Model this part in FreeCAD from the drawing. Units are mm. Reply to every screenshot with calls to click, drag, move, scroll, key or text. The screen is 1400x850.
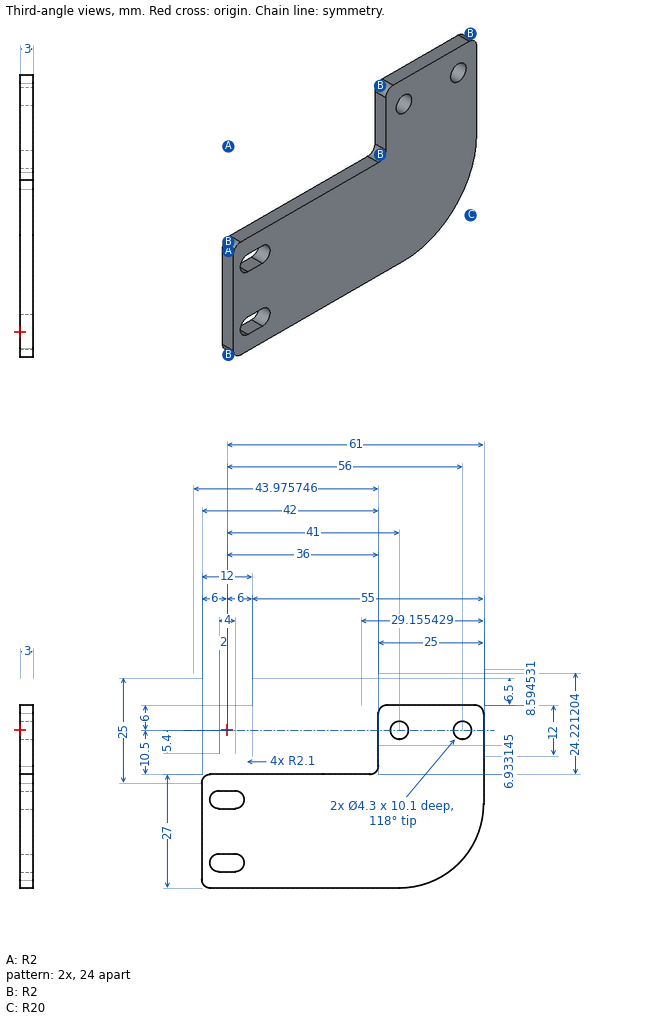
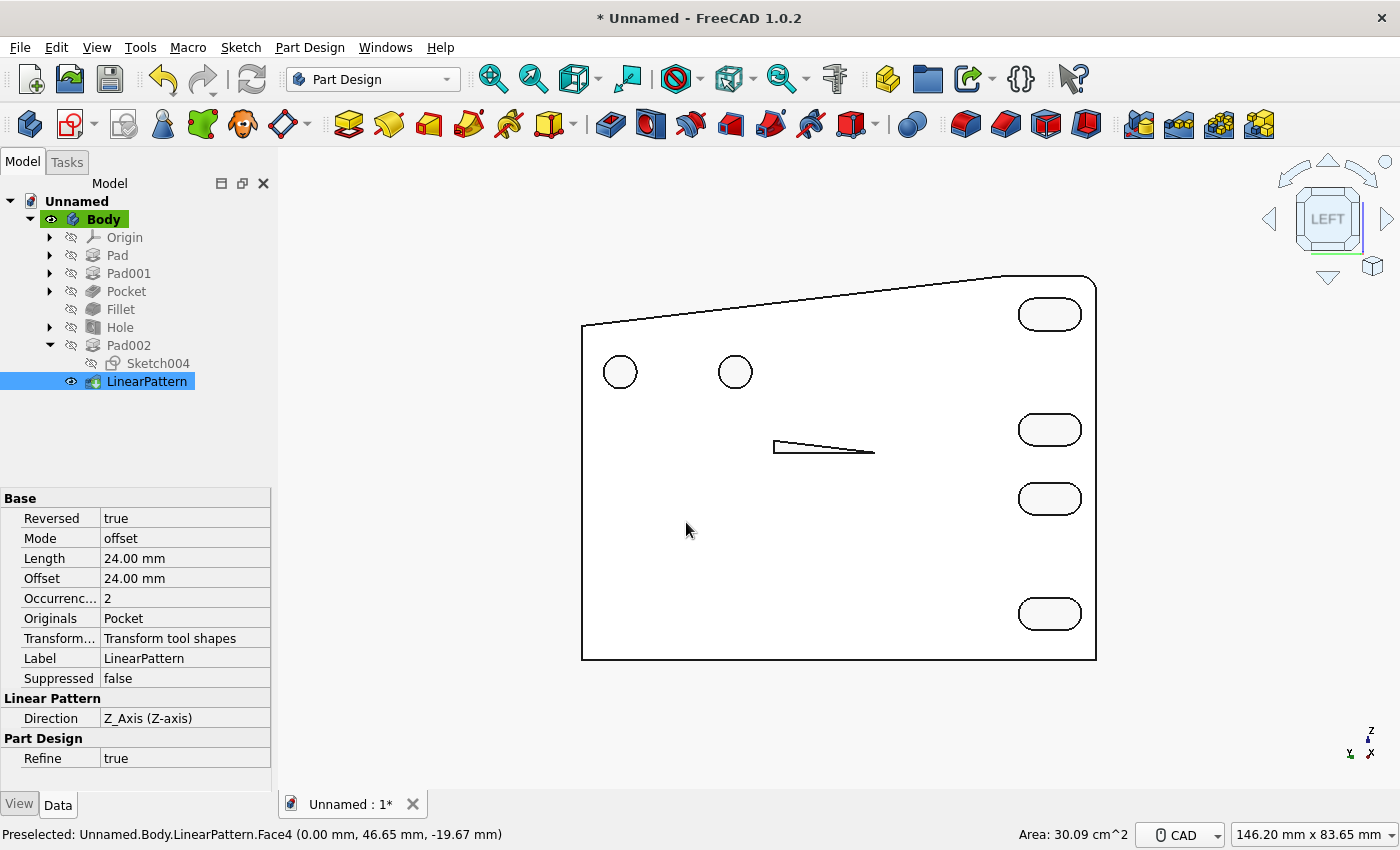
click(70, 124)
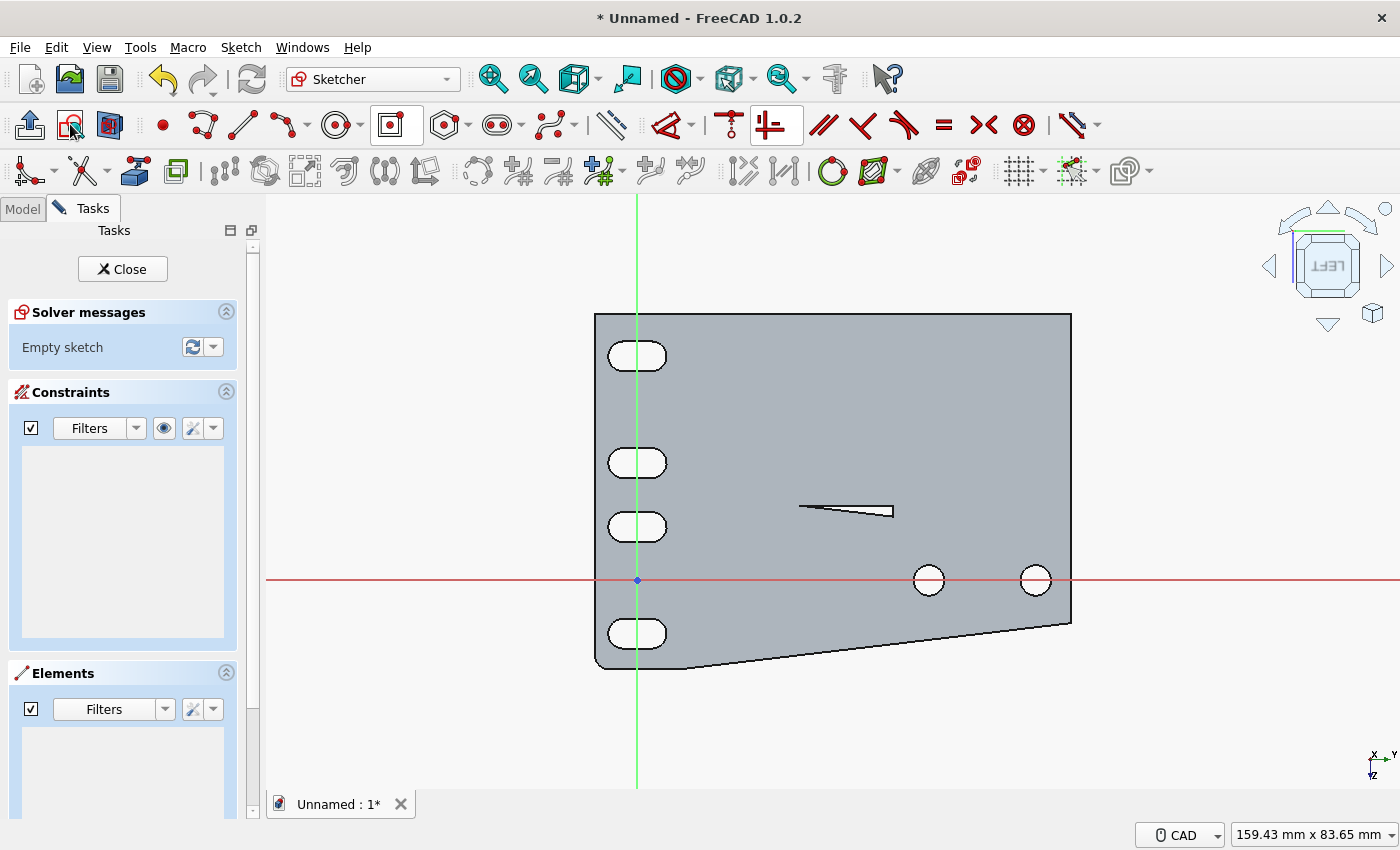
scroll(715, 674, up, 4)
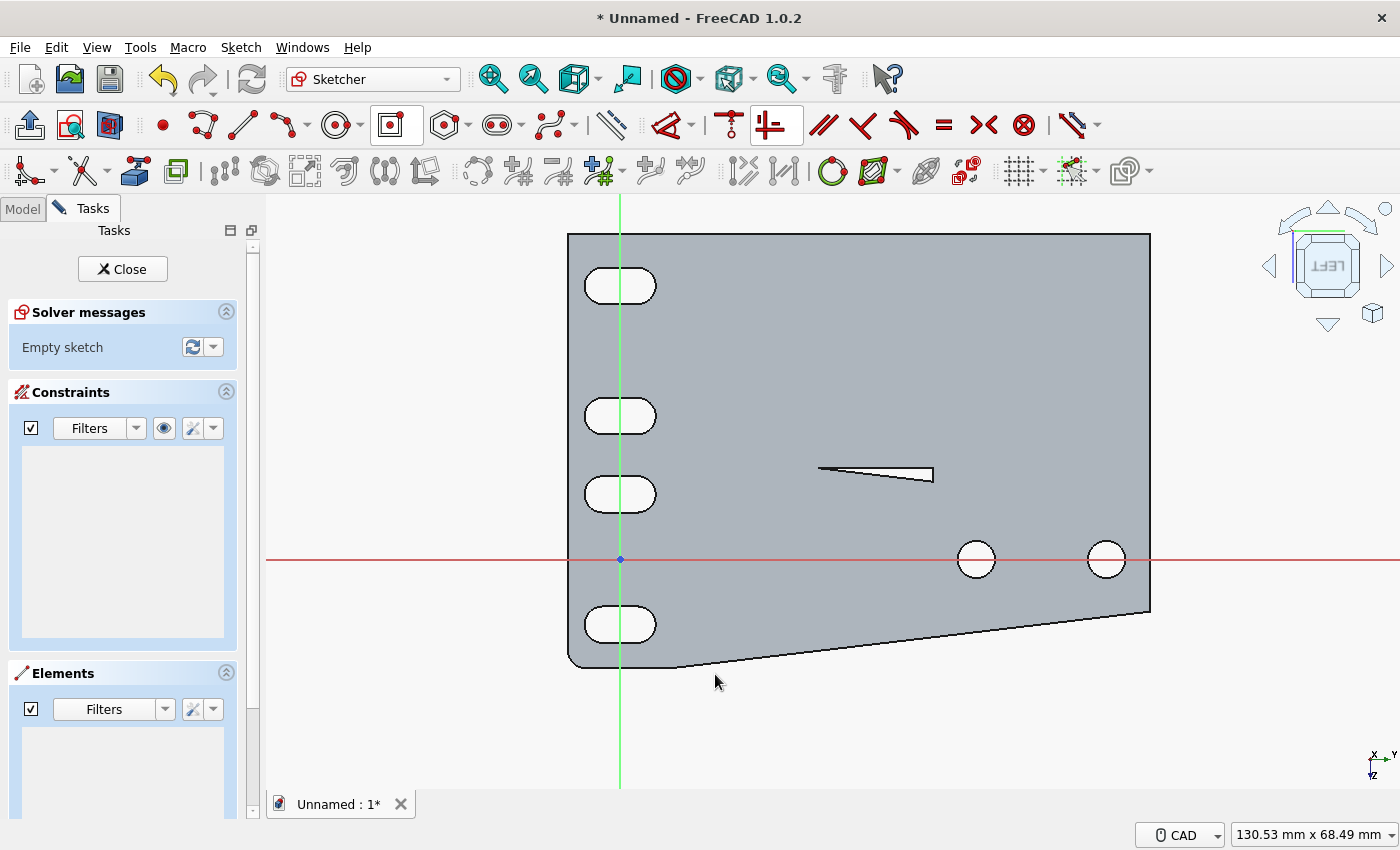
click(418, 126)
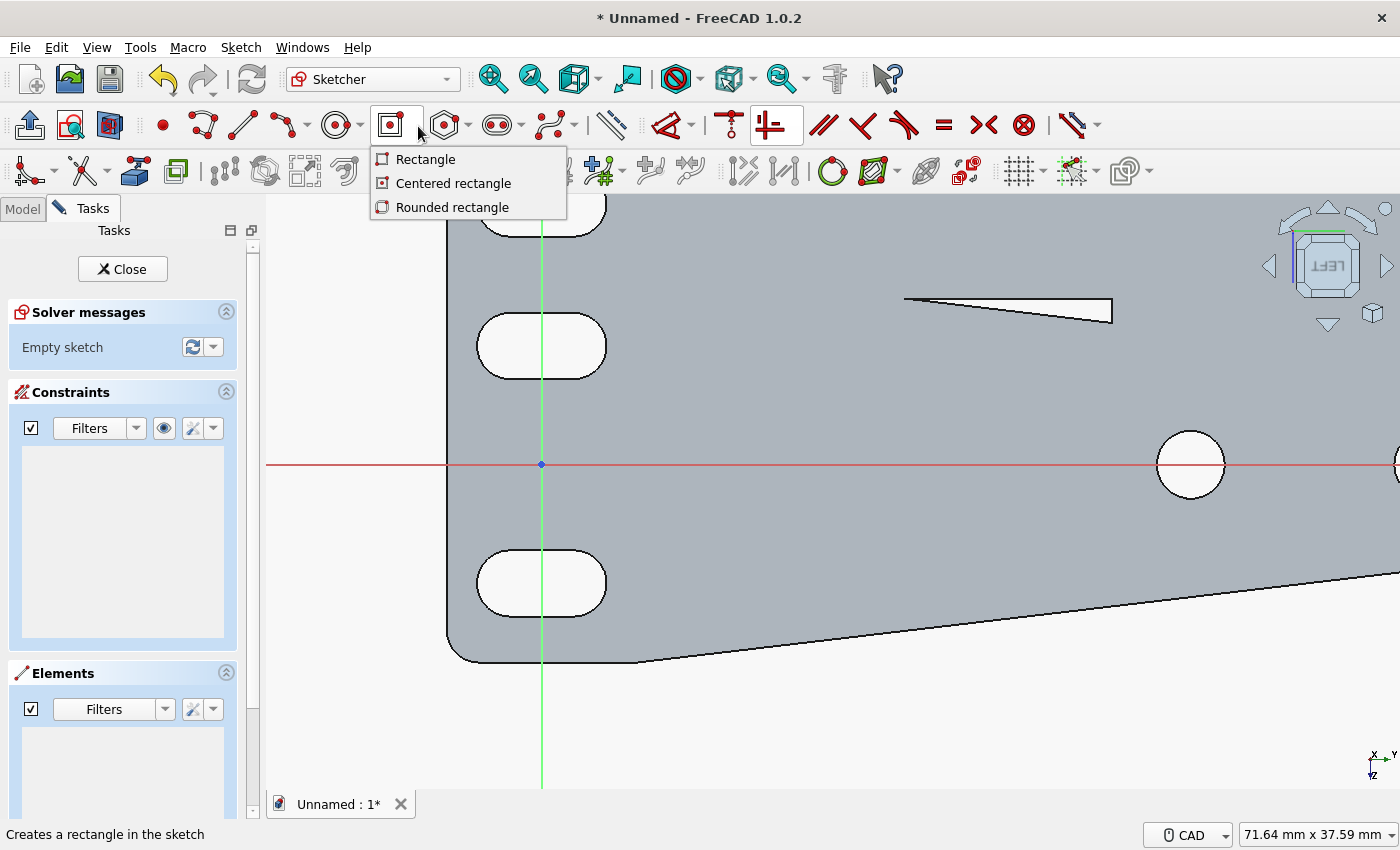
click(468, 159)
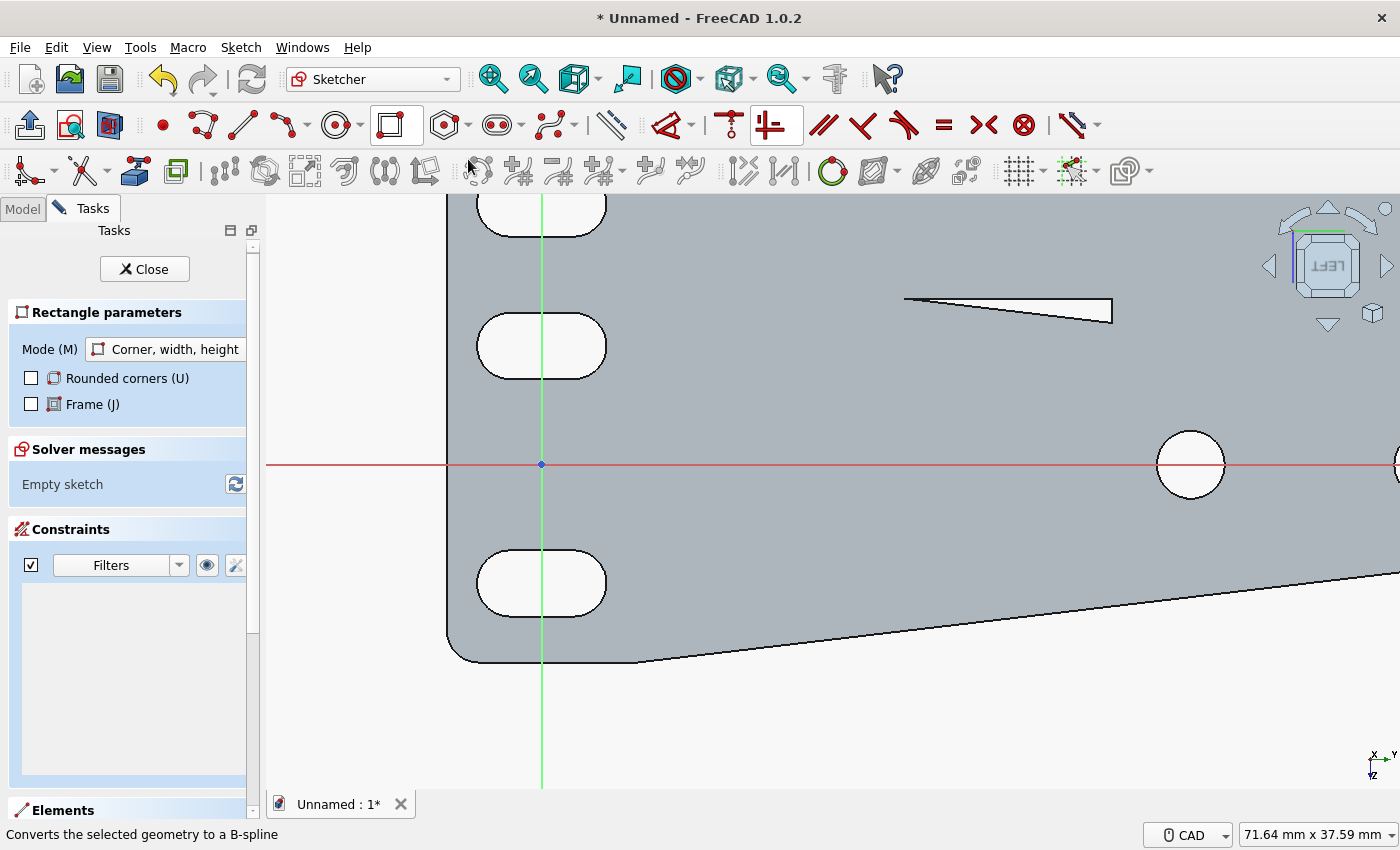
click(416, 299)
move(1112, 682)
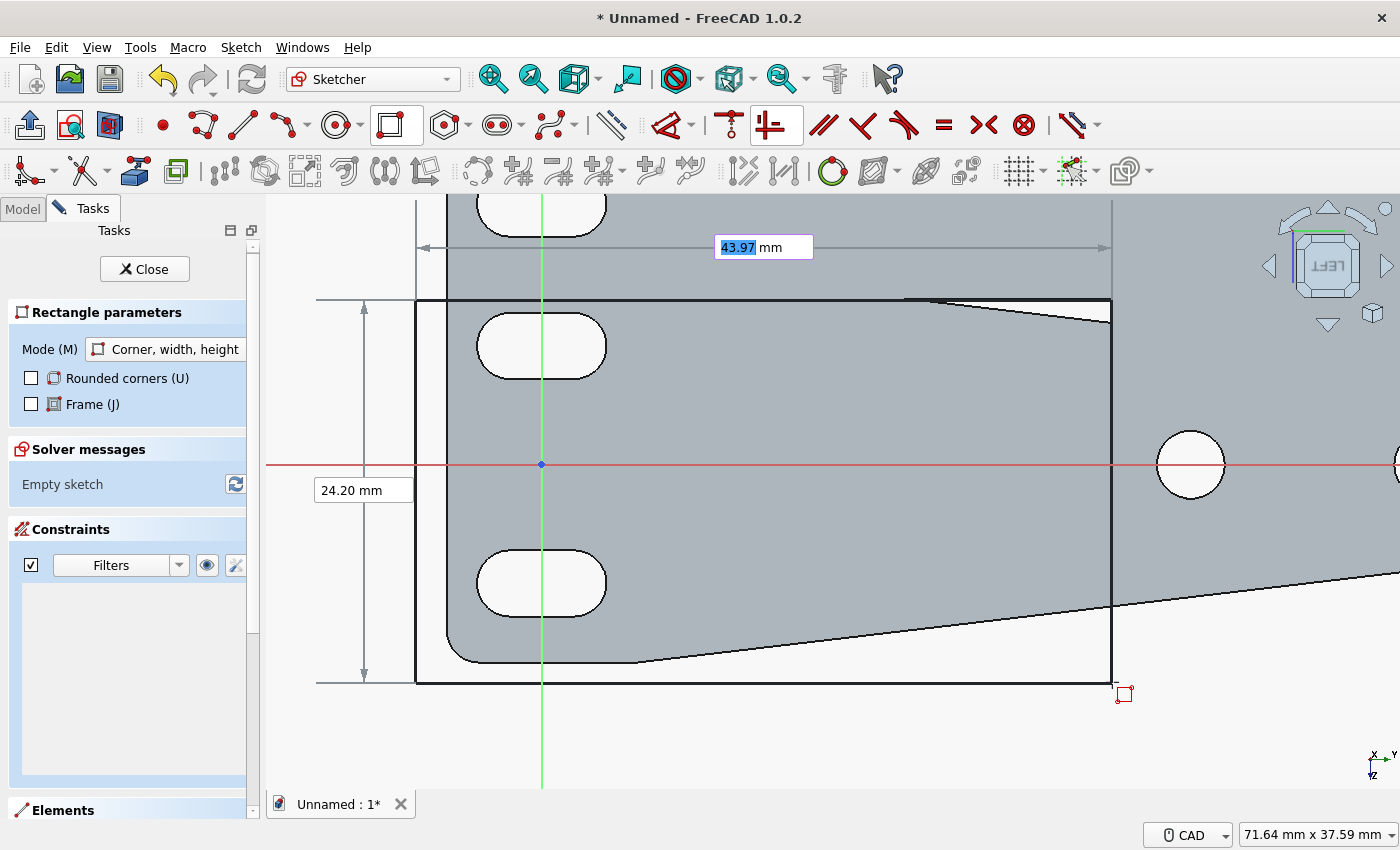
text(43.975746)
key(Tab)
text(24.221204)
key(Return)
key(Escape)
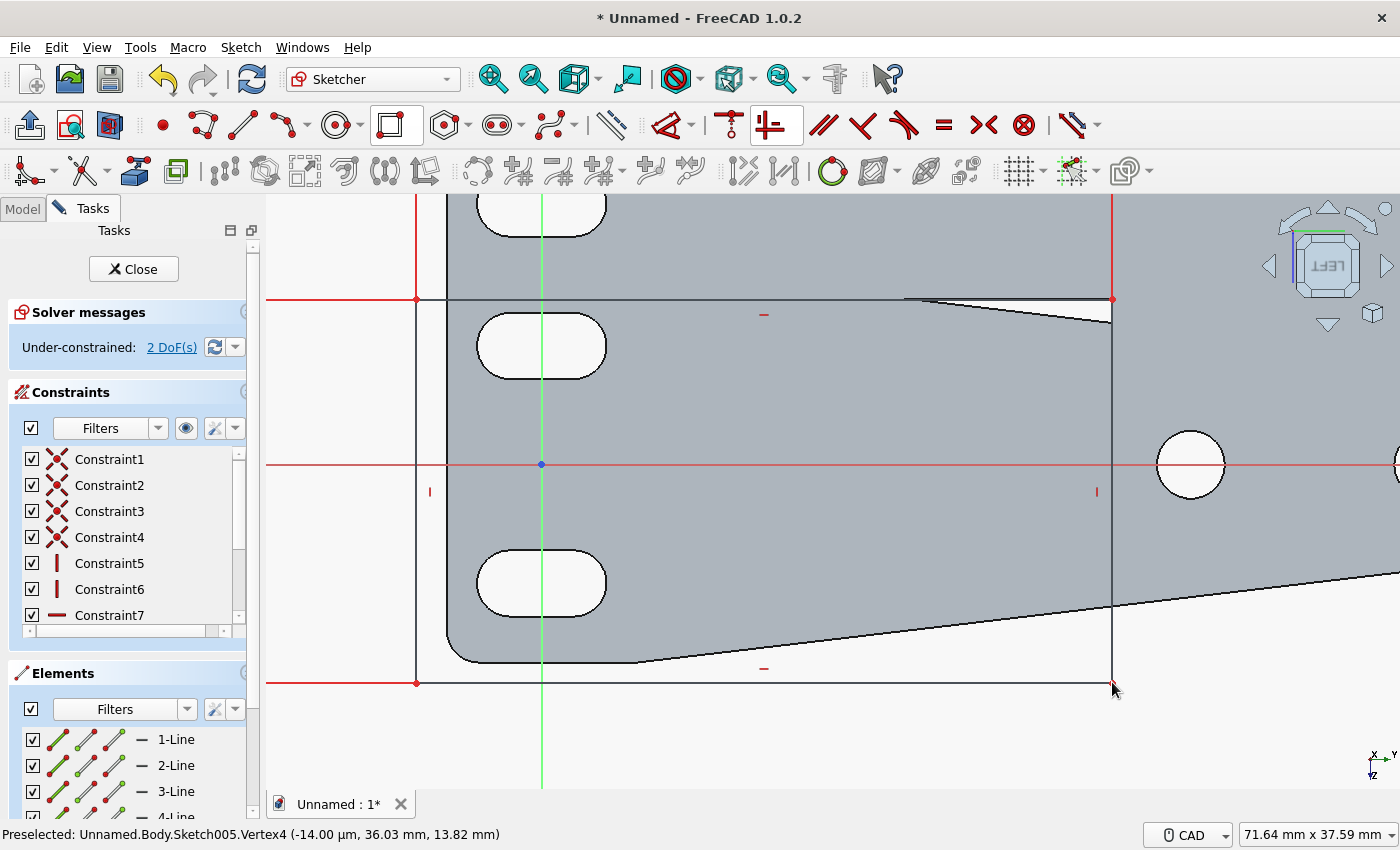
click(666, 126)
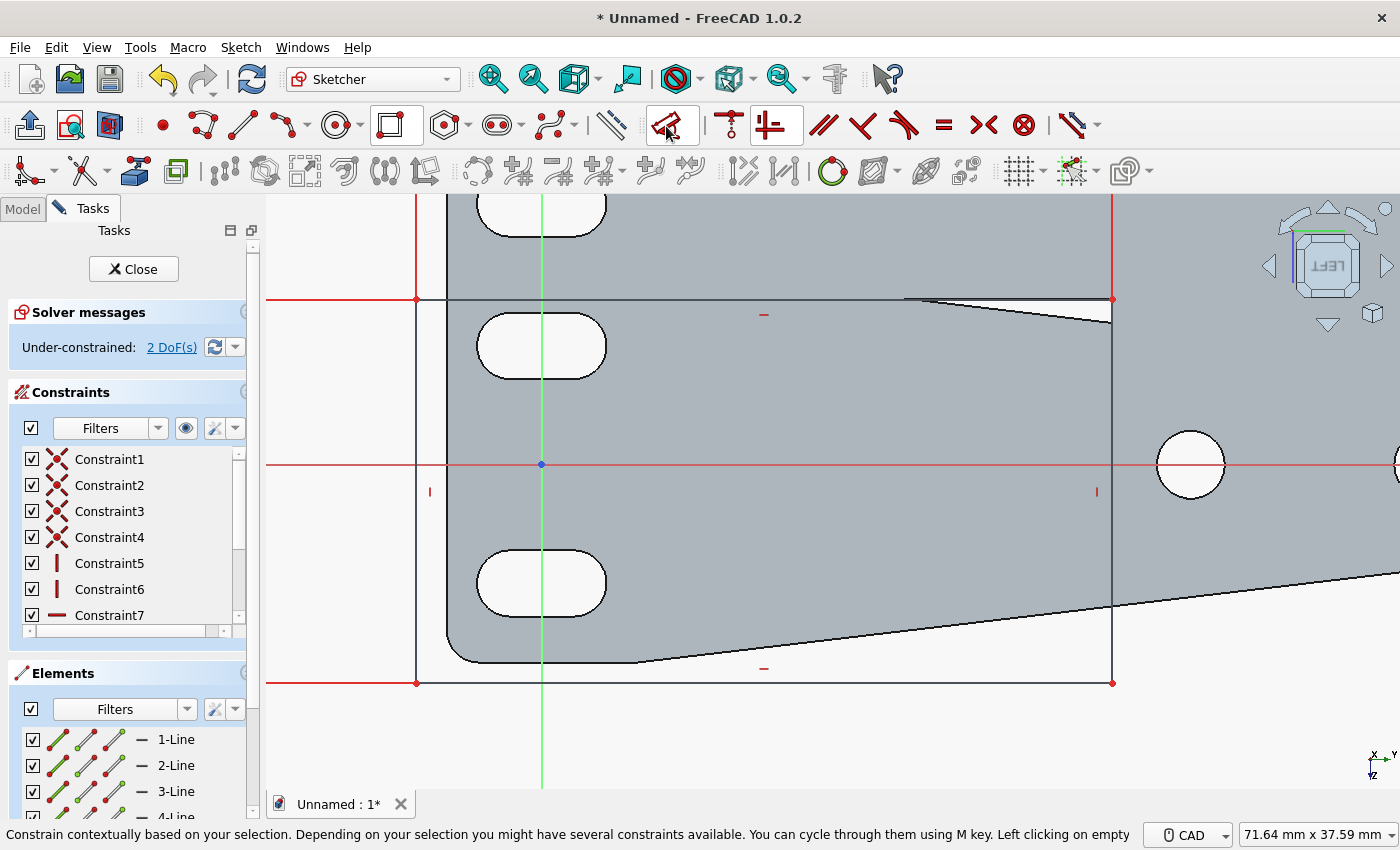
click(1112, 683)
click(827, 717)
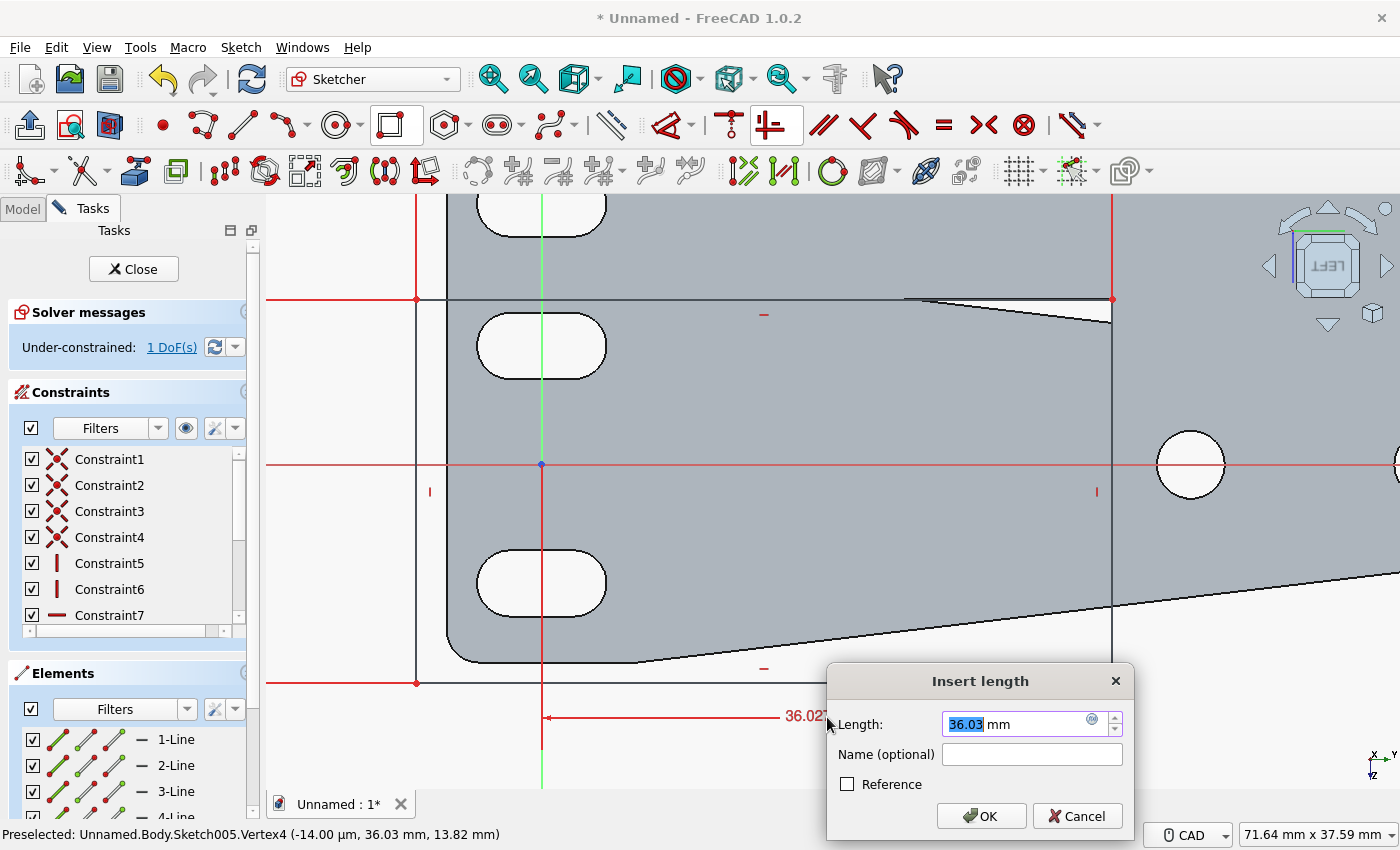
text(36)
key(Return)